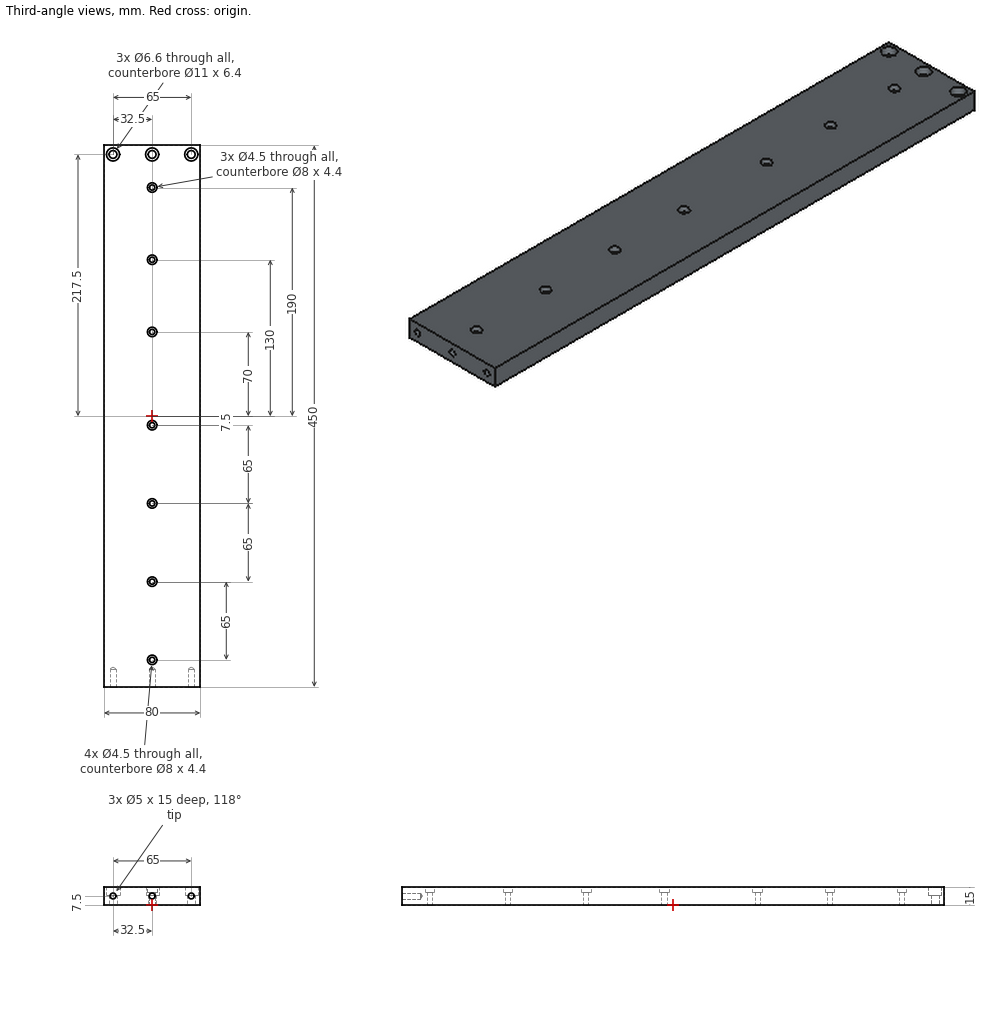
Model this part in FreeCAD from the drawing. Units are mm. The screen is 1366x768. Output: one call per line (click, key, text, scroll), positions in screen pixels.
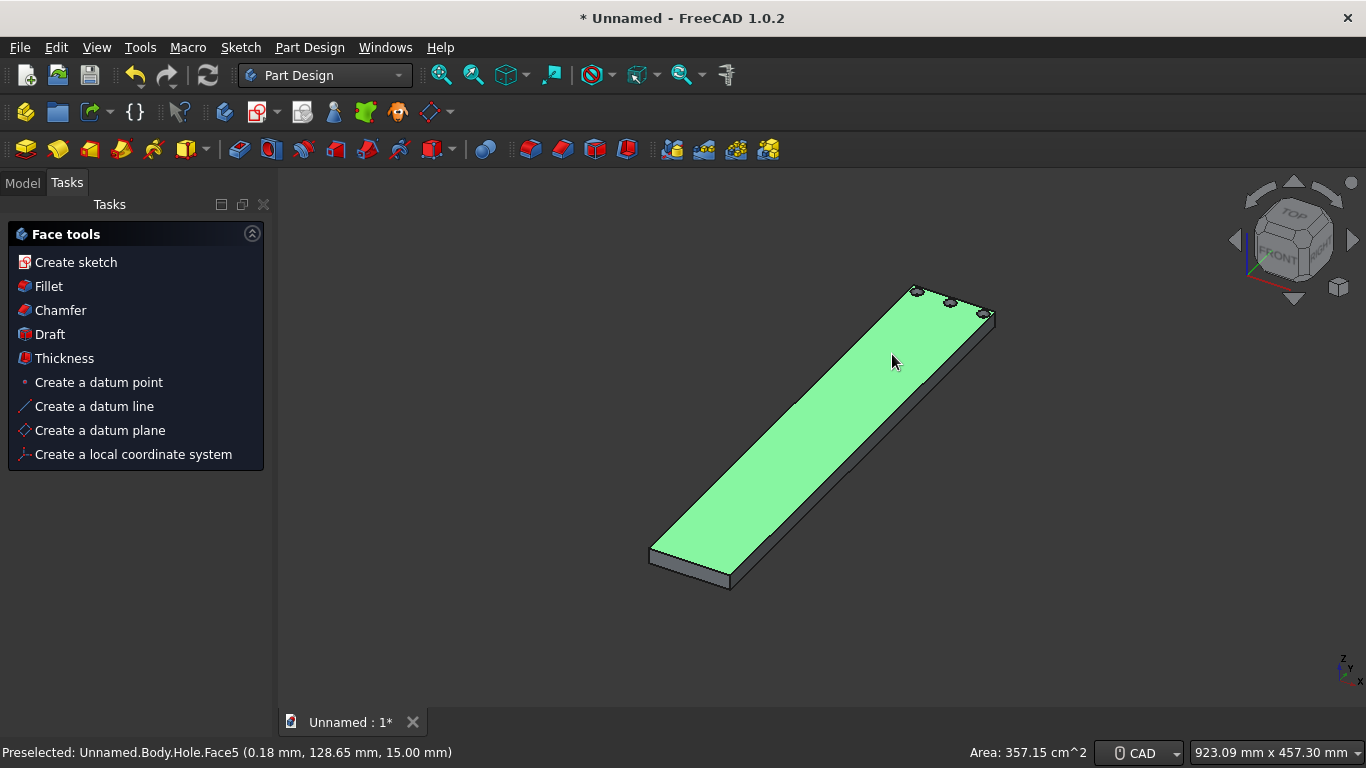
click(258, 112)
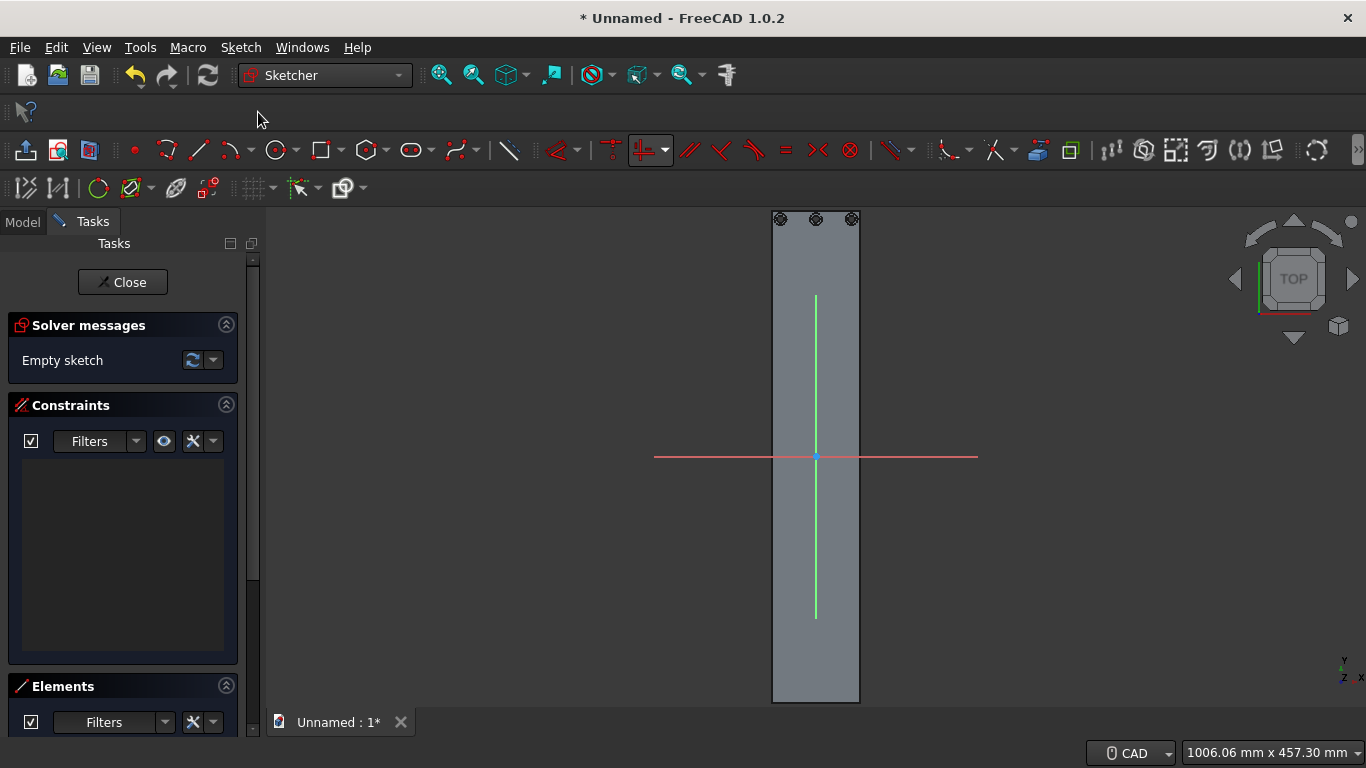
scroll(438, 679, down, 1)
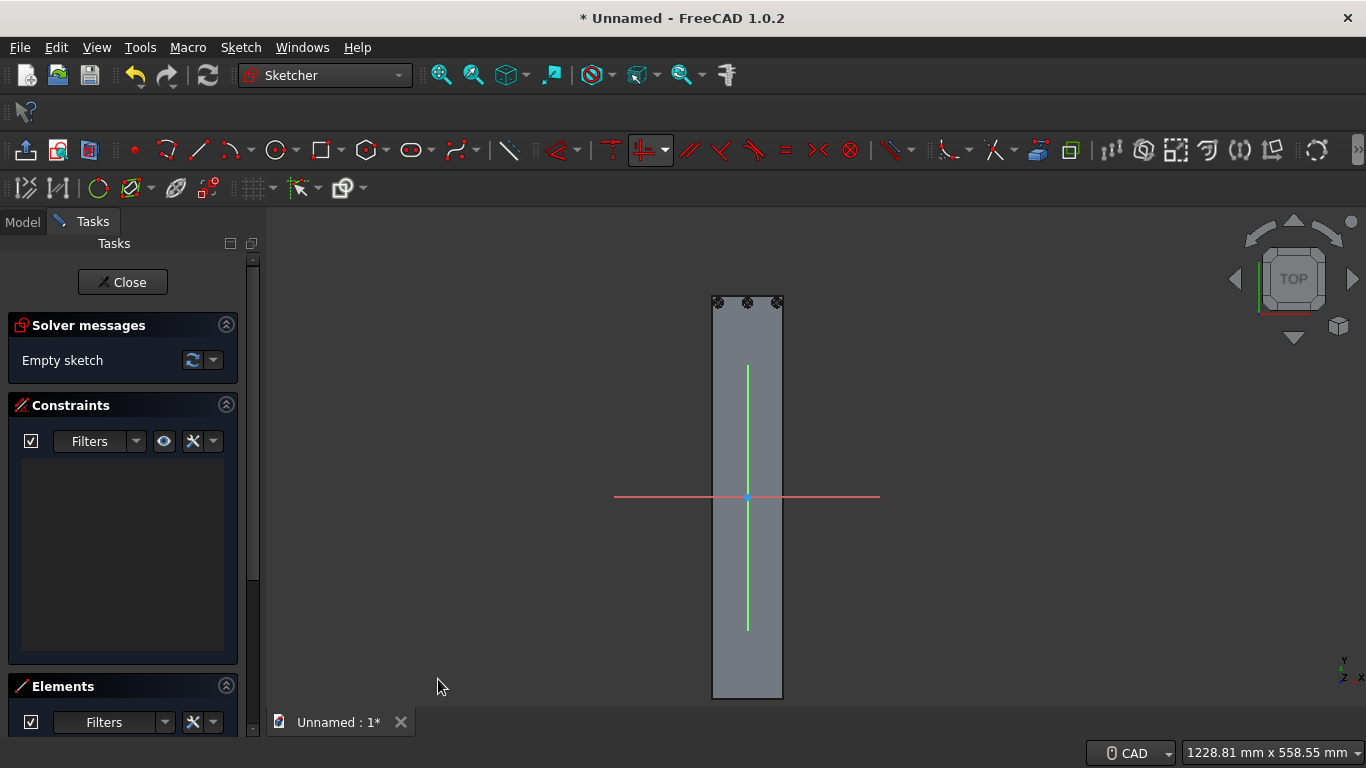
scroll(748, 356, up, 3)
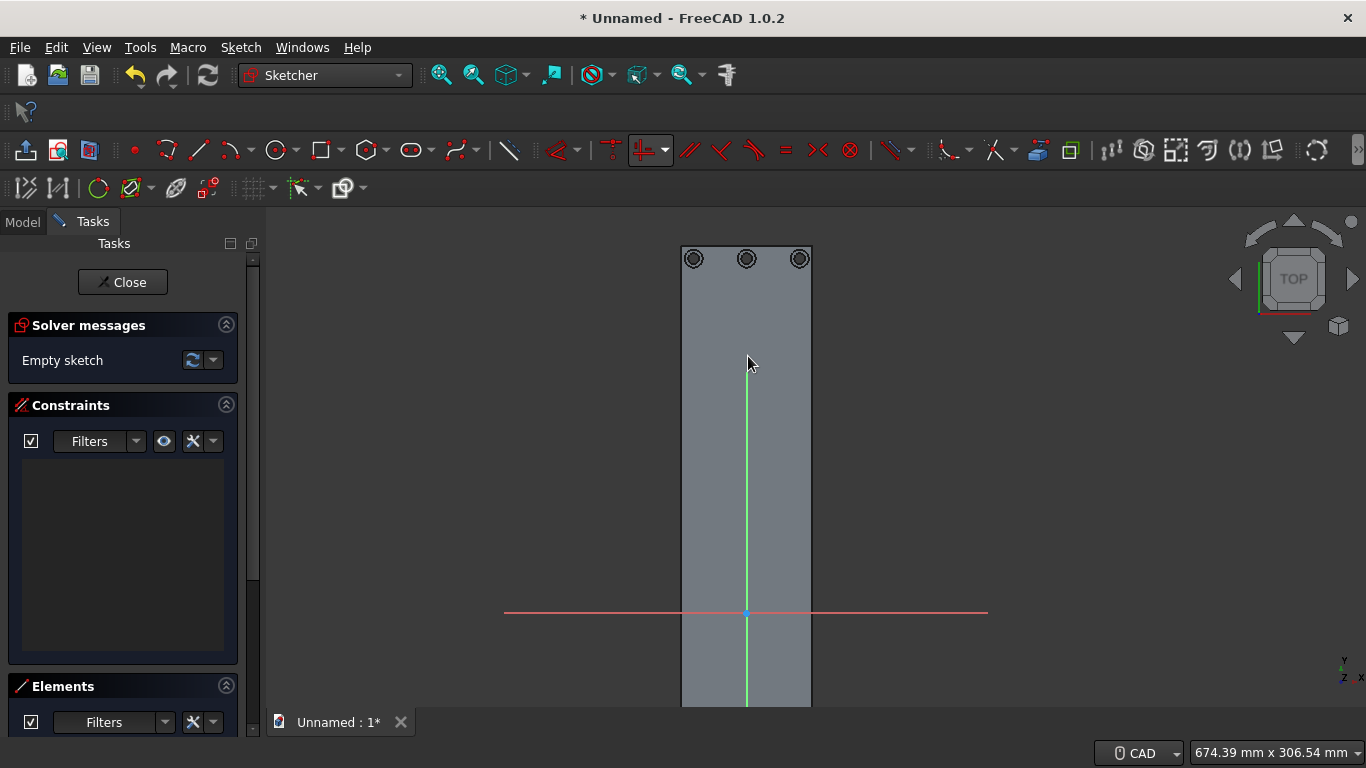
click(276, 150)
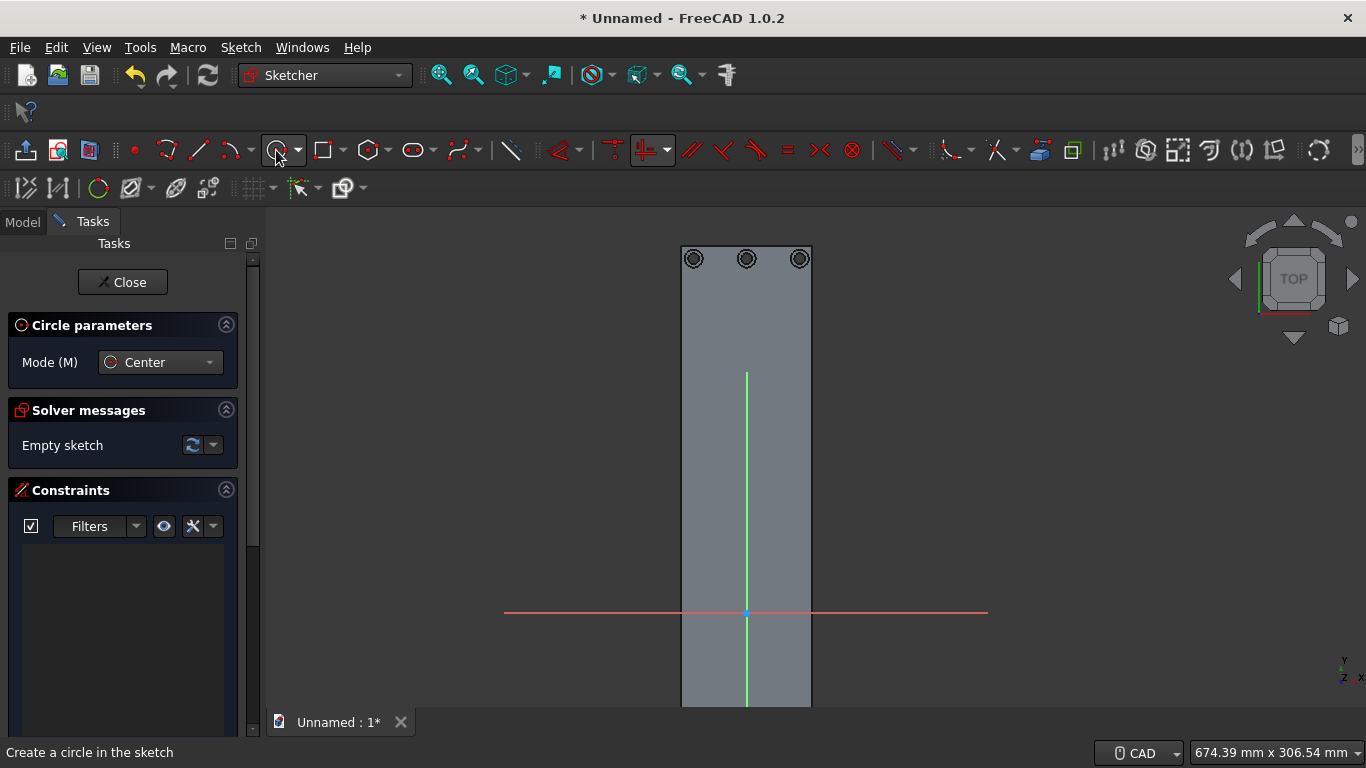
scroll(747, 304, up, 10)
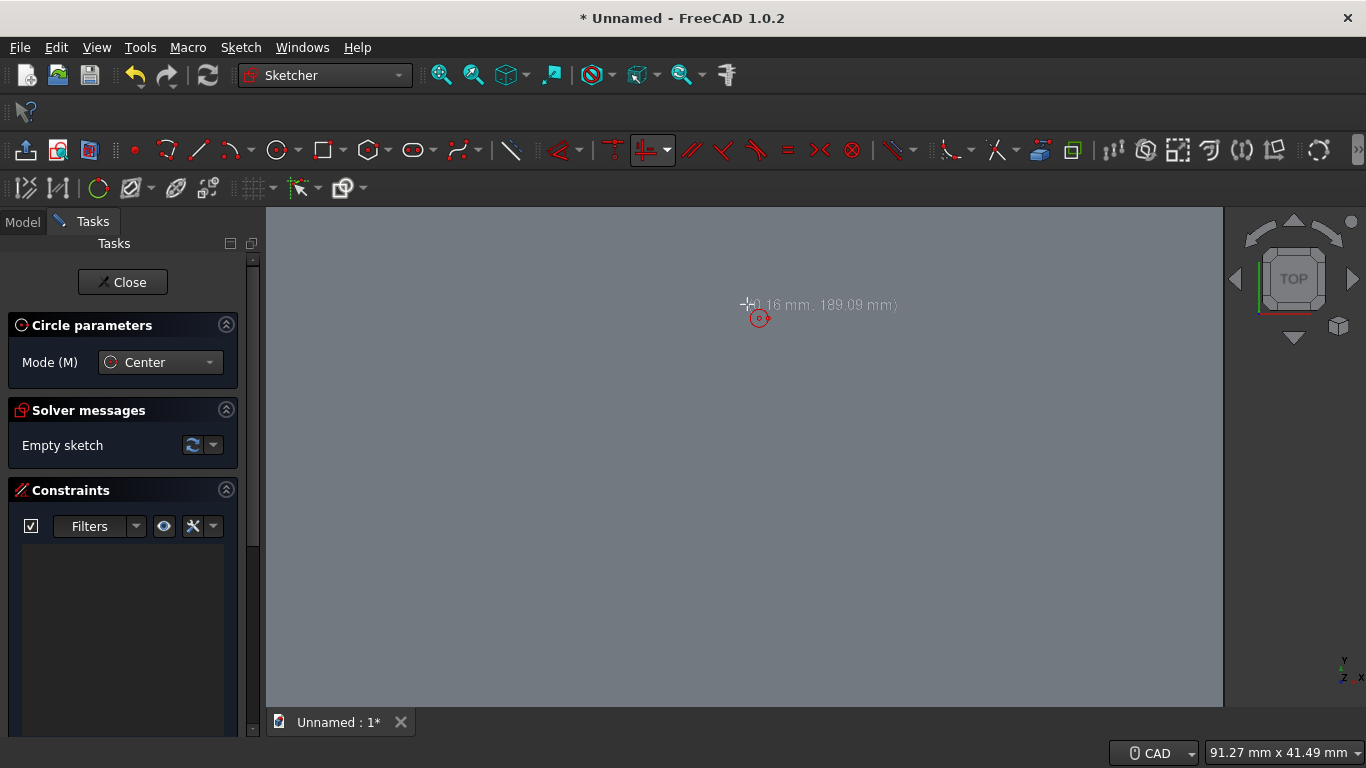
scroll(748, 305, down, 10)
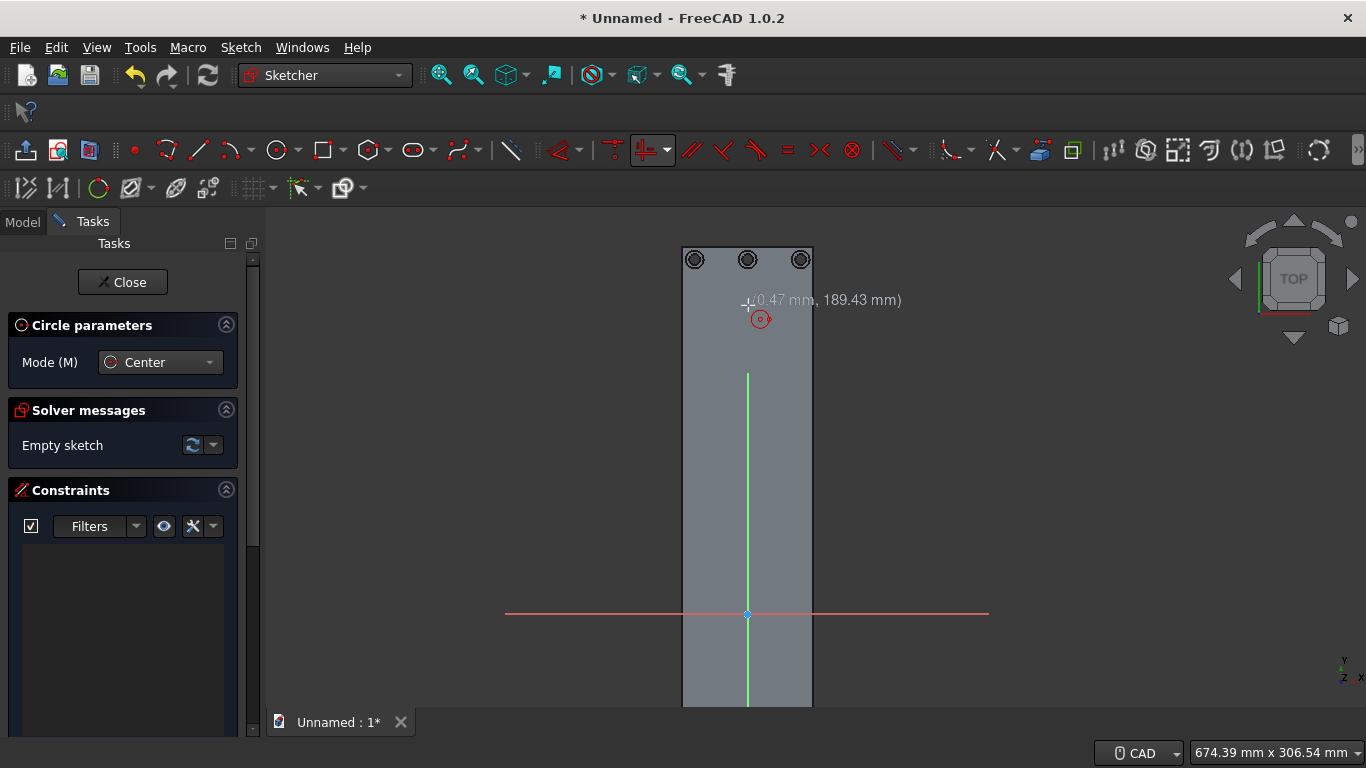
click(748, 304)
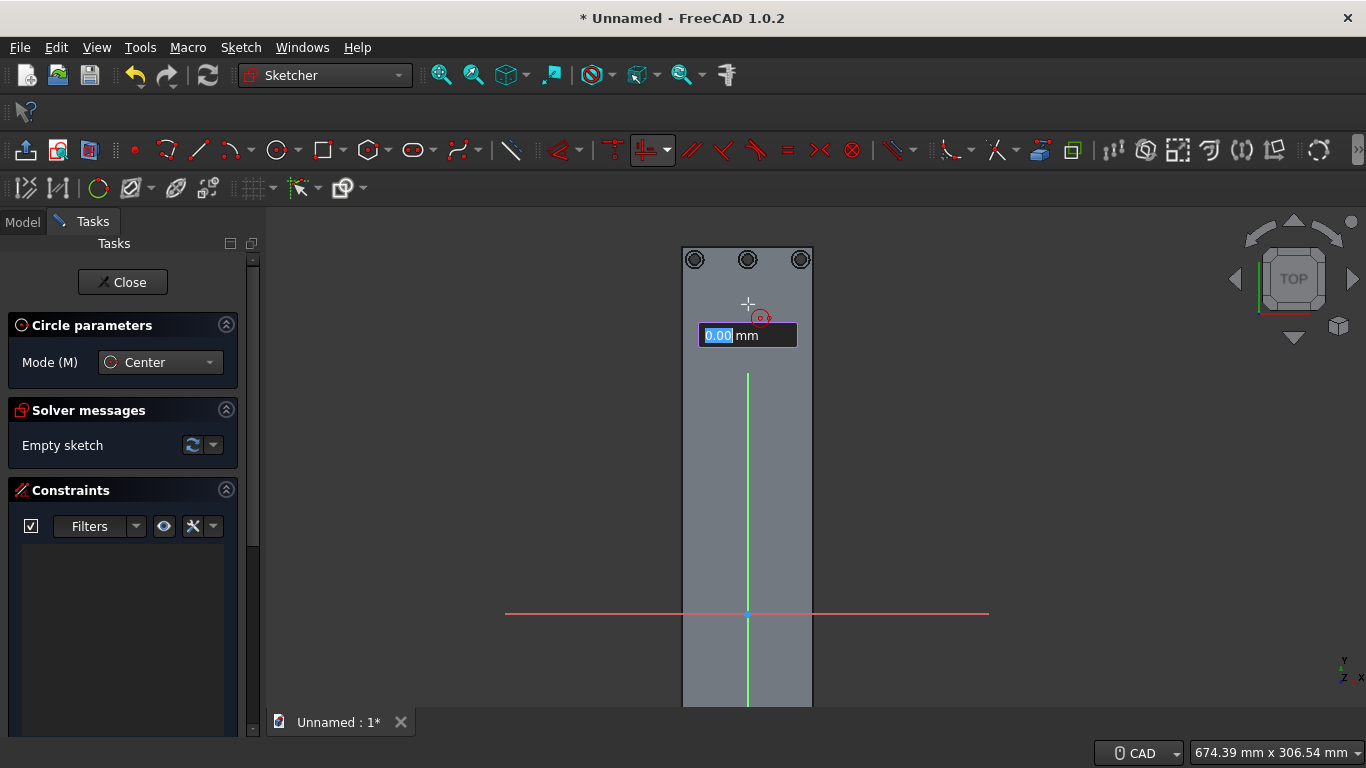
scroll(751, 303, up, 8)
move(750, 303)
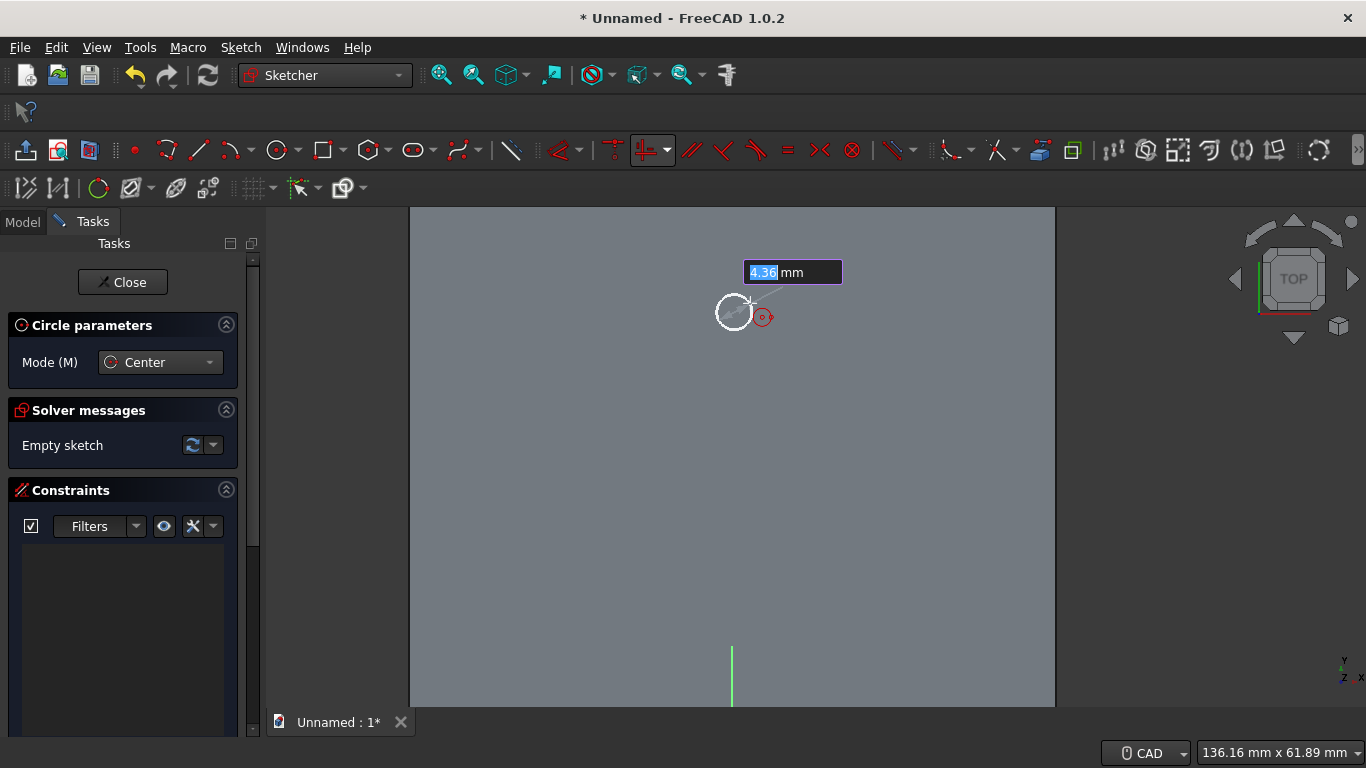
text(4.5)
key(Return)